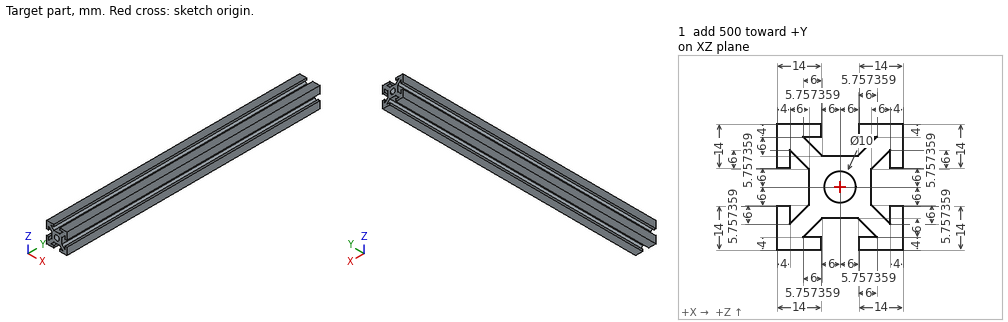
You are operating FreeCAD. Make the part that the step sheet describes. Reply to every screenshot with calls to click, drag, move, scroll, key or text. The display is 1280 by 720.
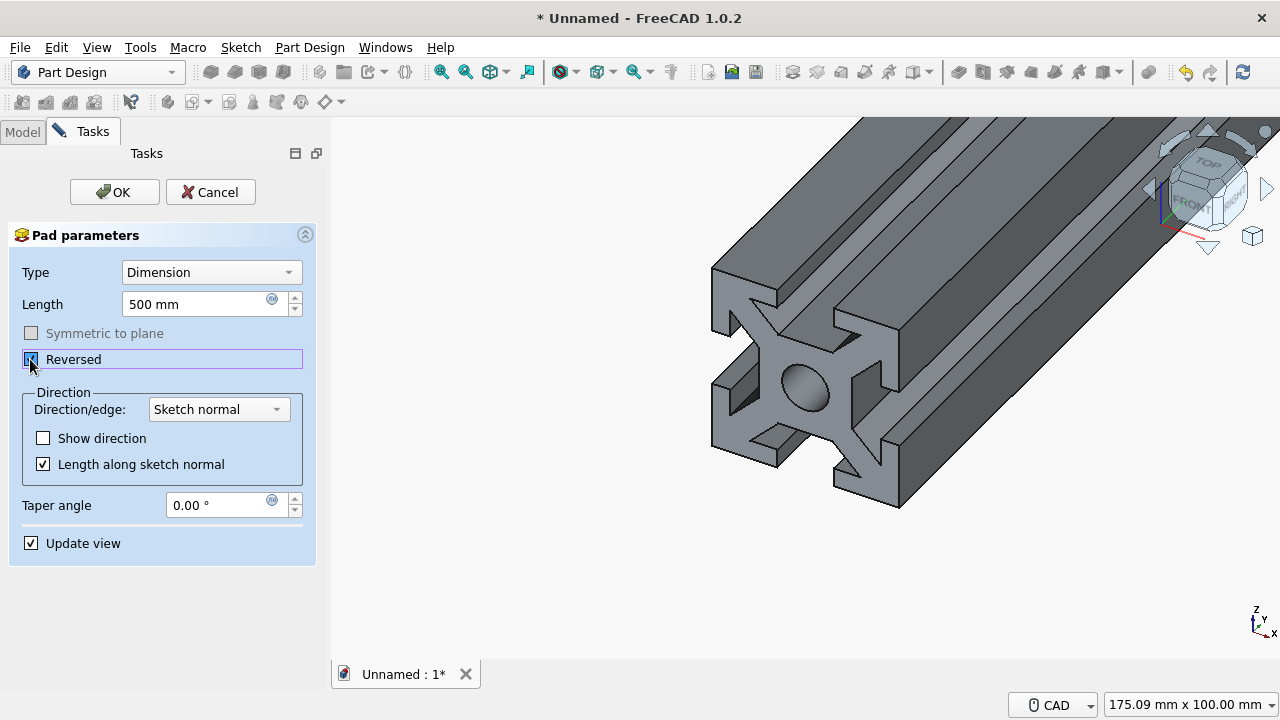
click(115, 192)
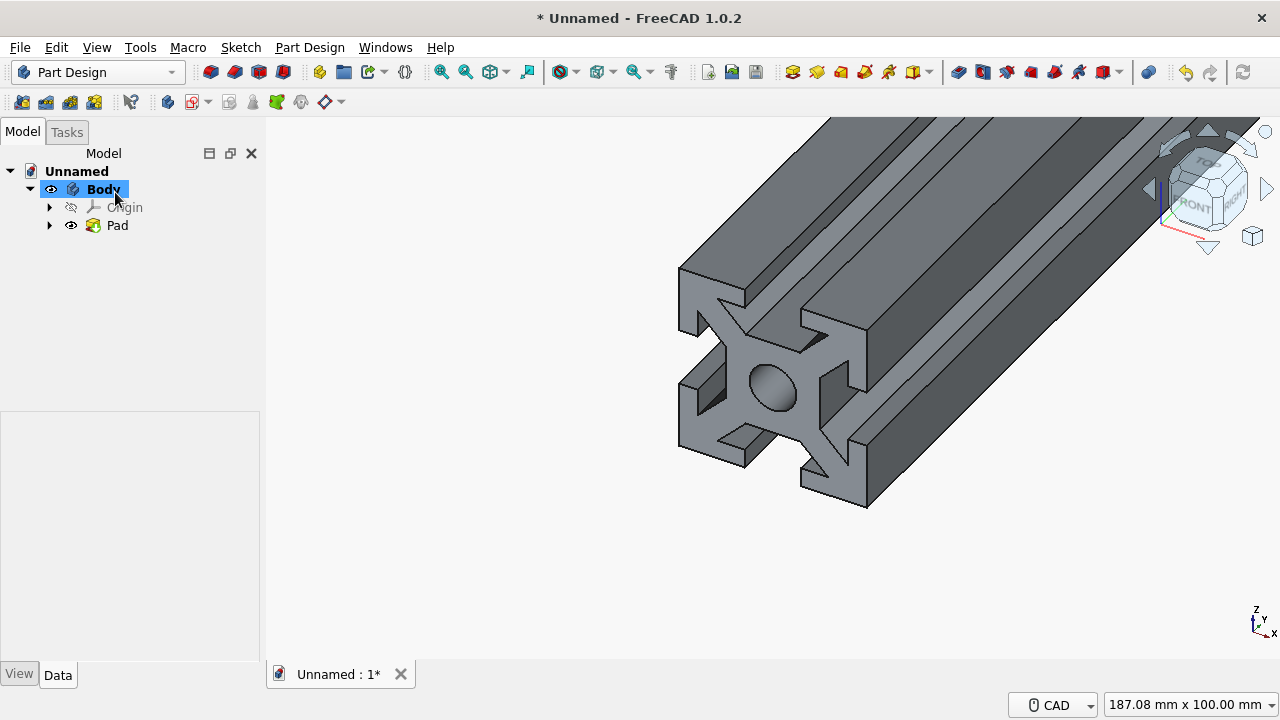
key(0)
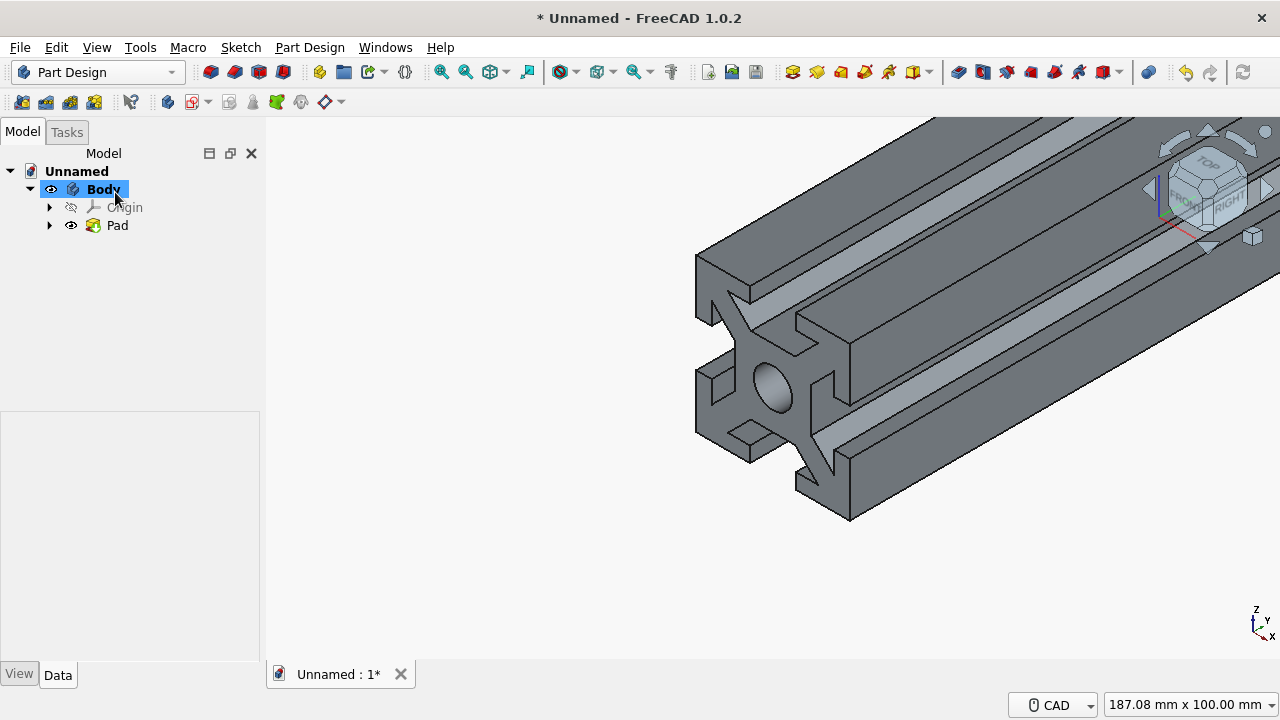
click(442, 72)